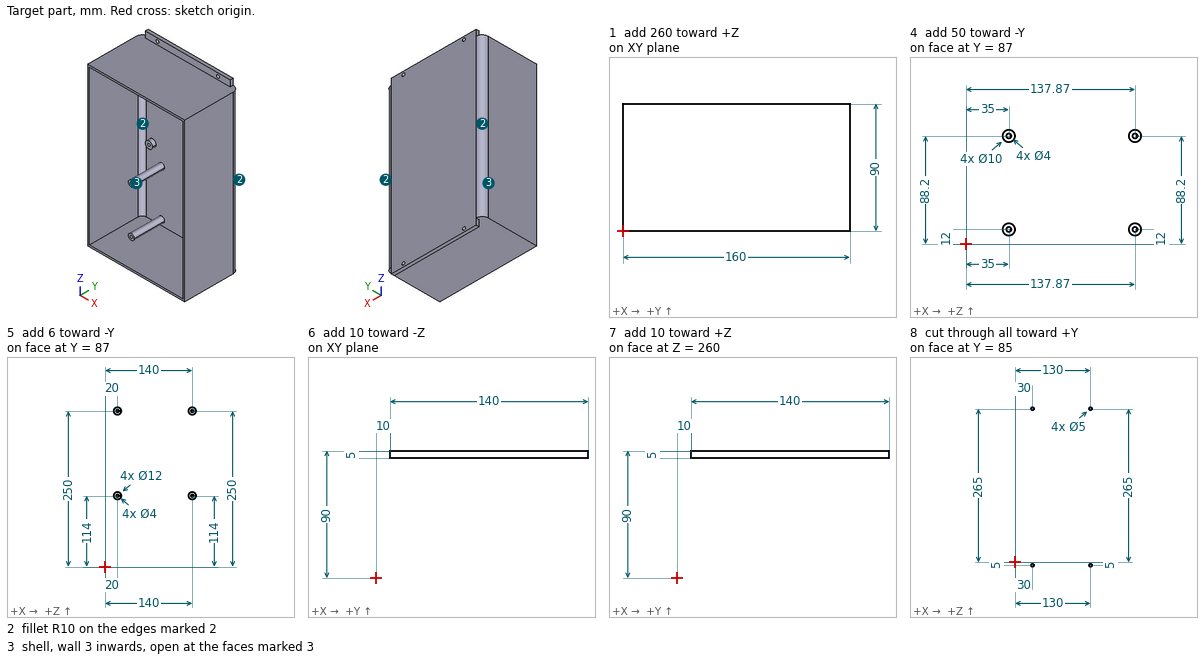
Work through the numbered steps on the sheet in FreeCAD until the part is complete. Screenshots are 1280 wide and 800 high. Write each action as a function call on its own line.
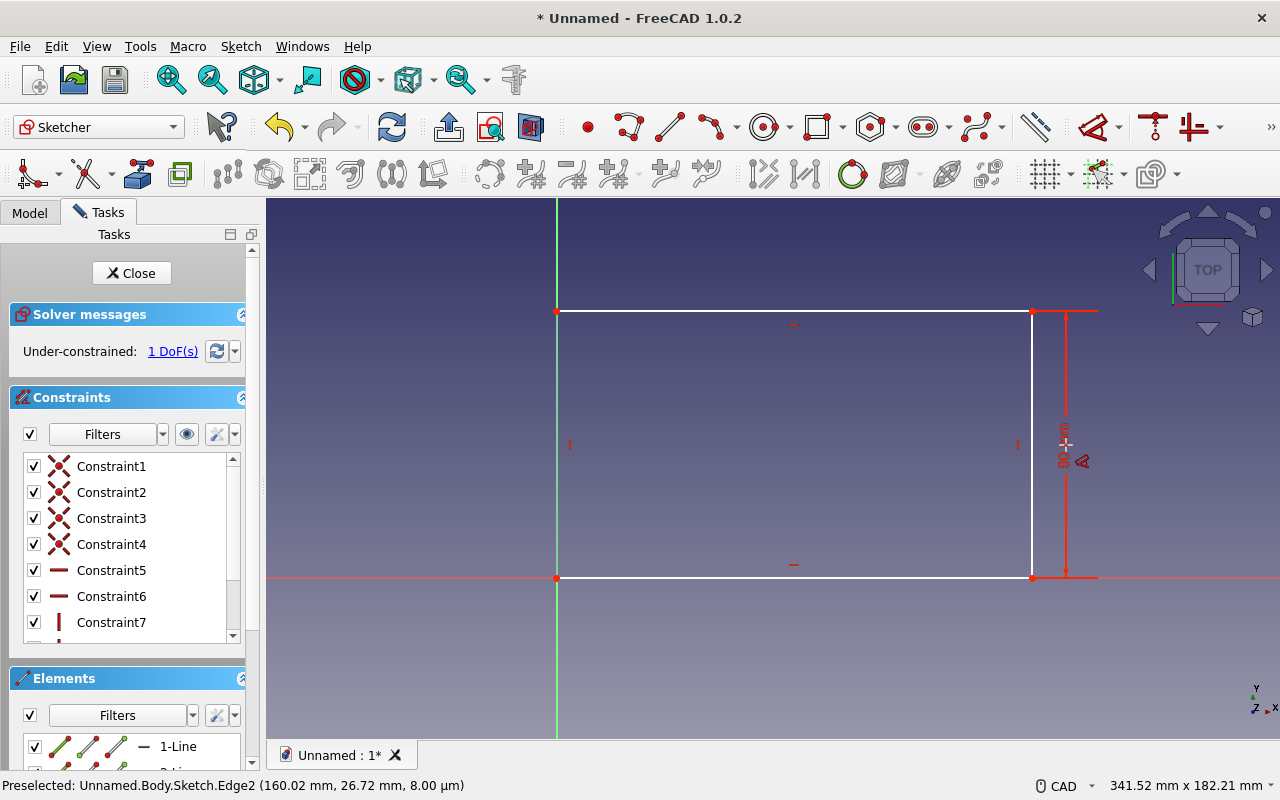
click(699, 578)
click(794, 612)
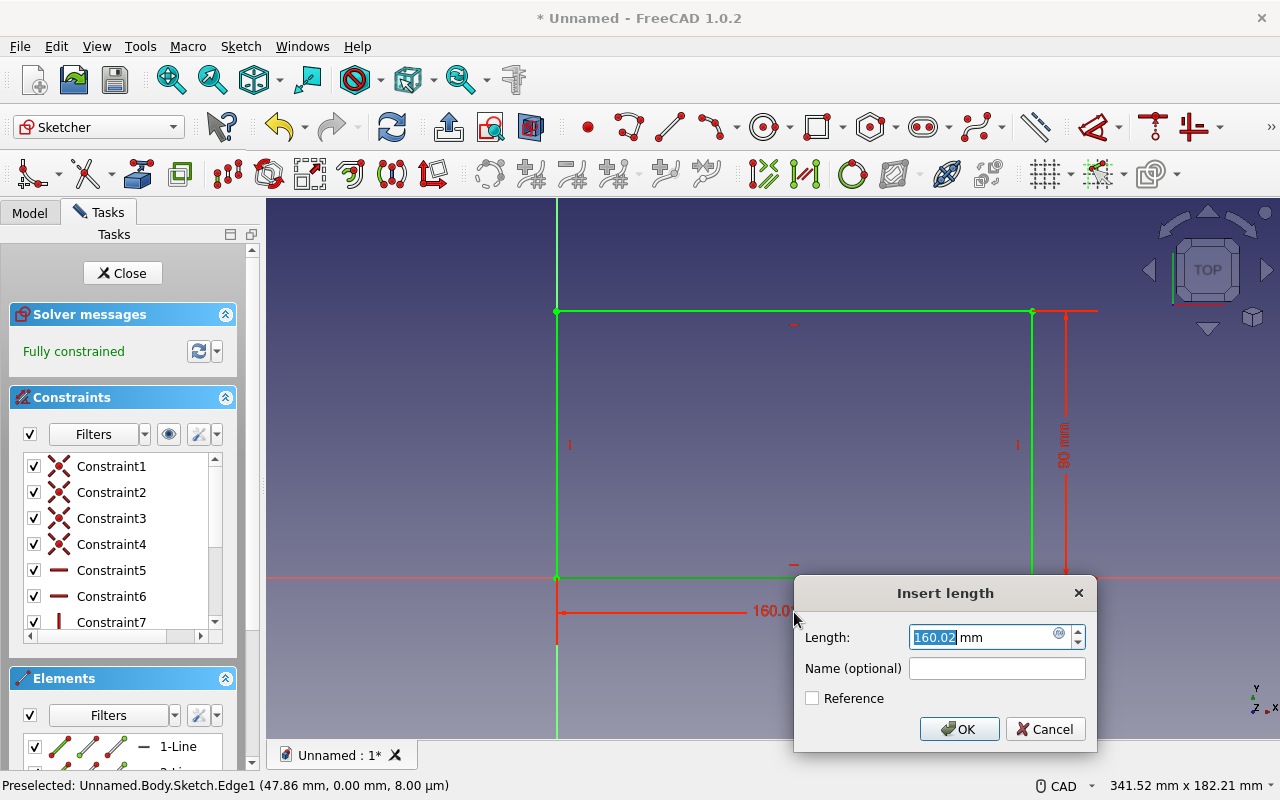
text(160)
key(Return)
key(Escape)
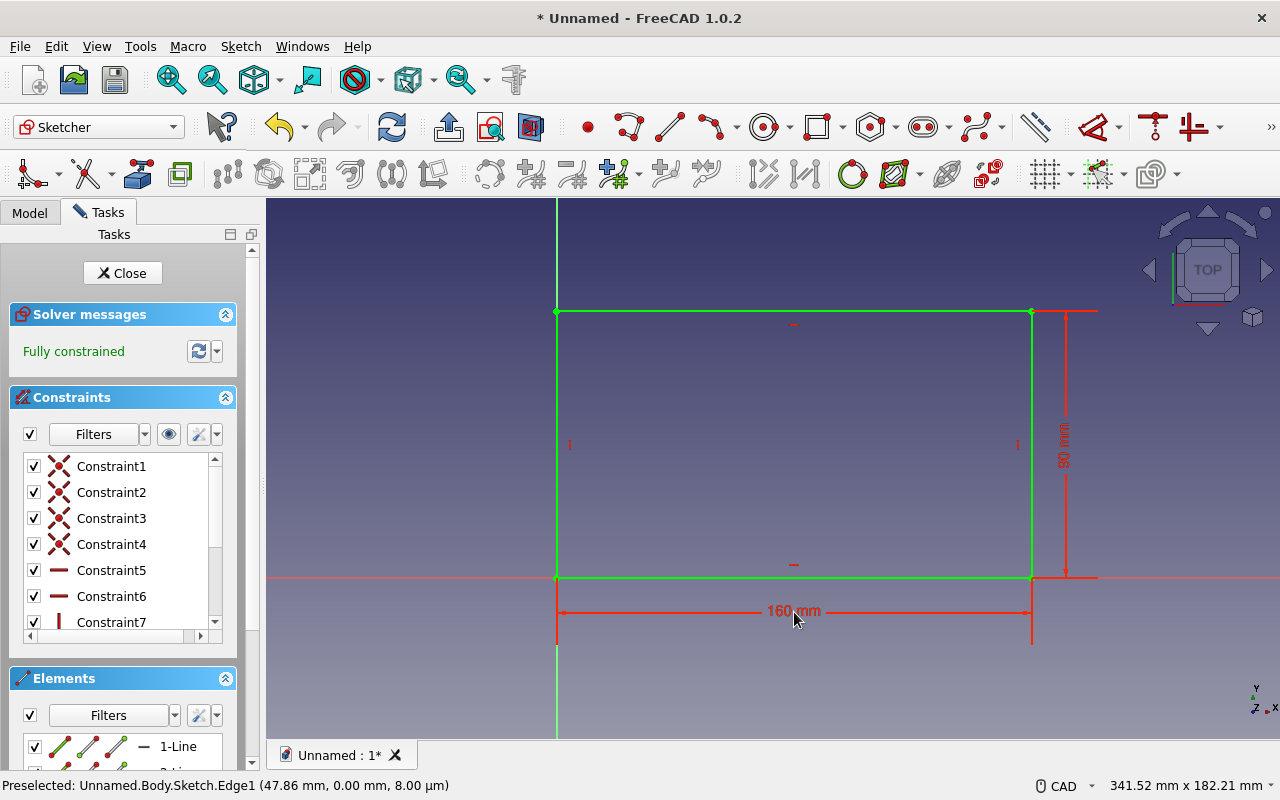
click(123, 273)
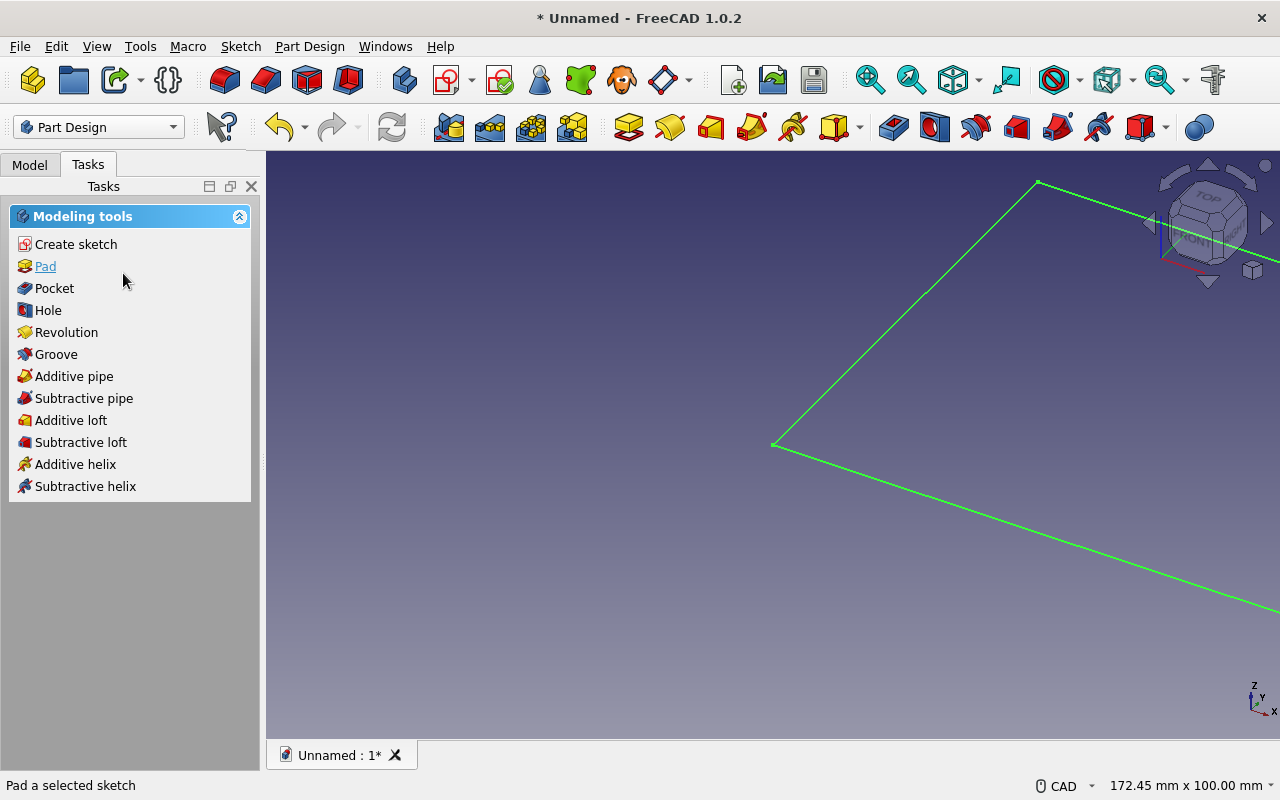
click(629, 128)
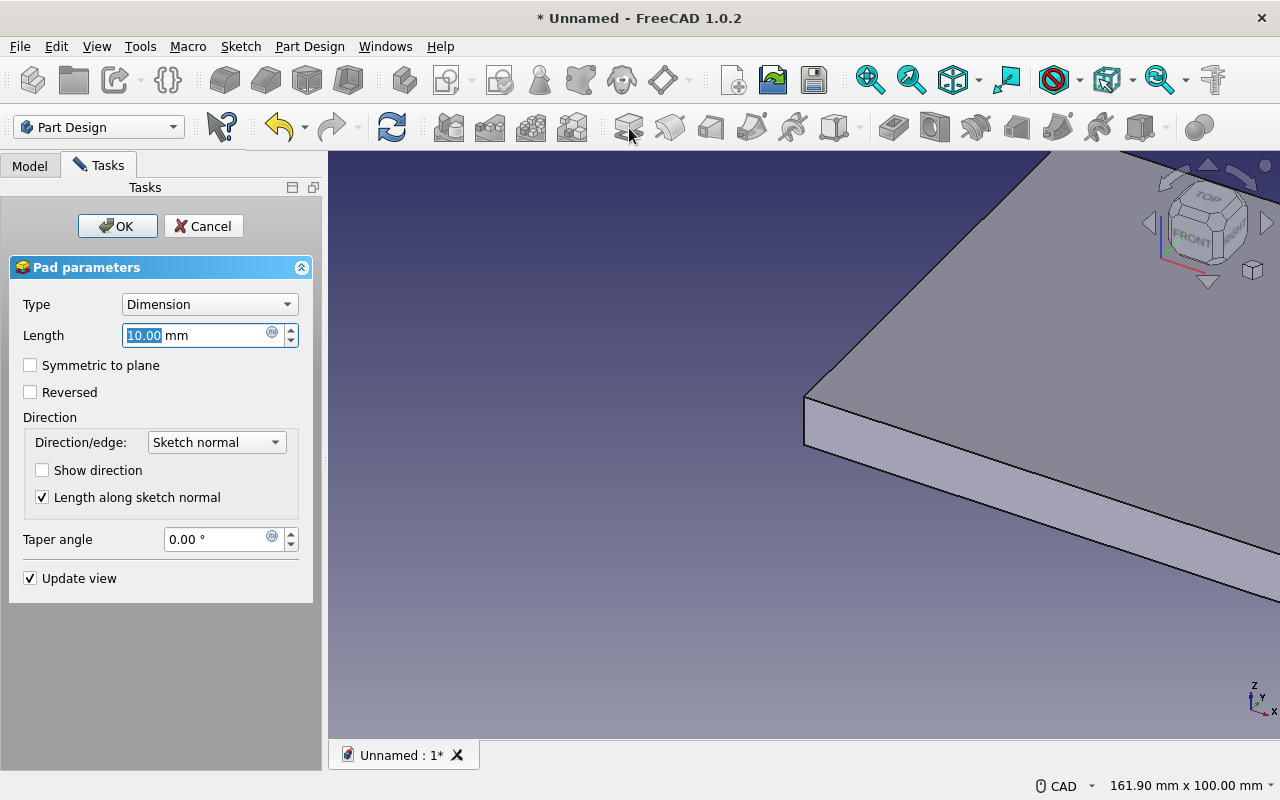
text(260)
key(Tab)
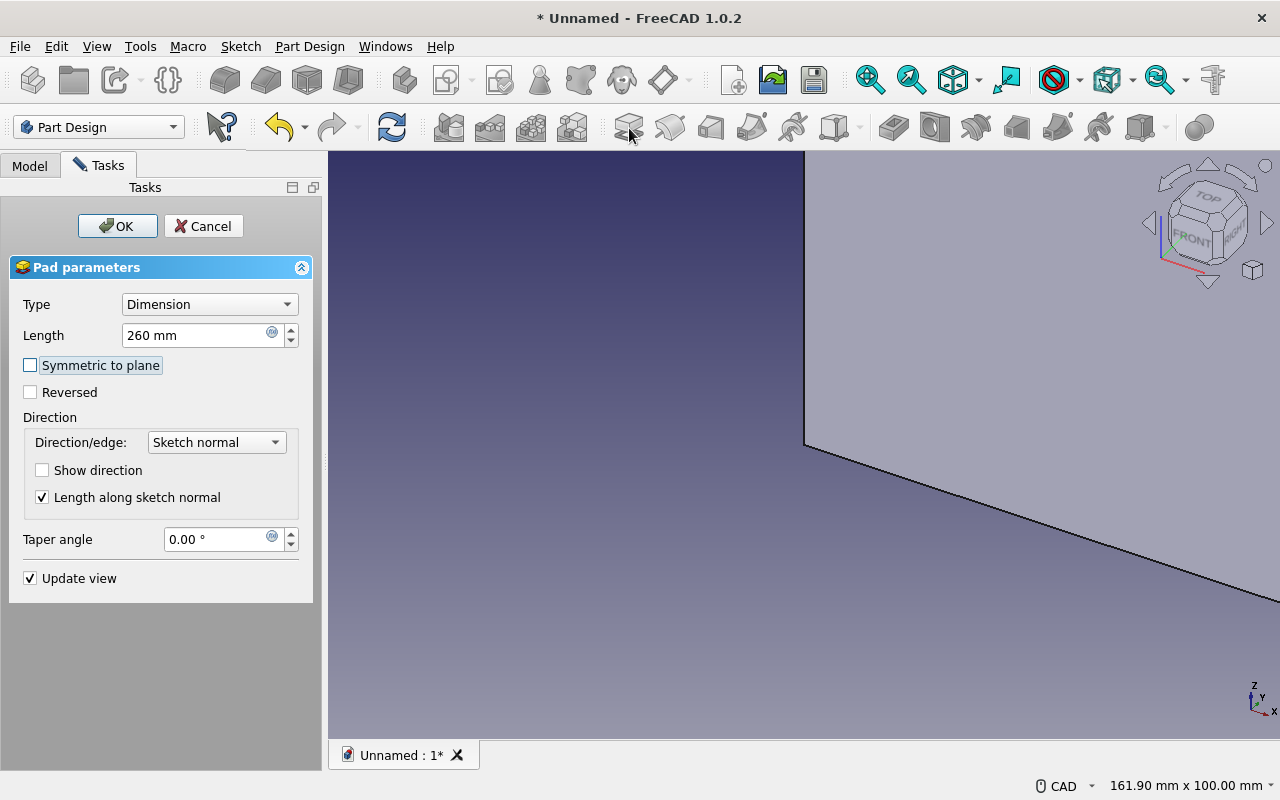
click(118, 226)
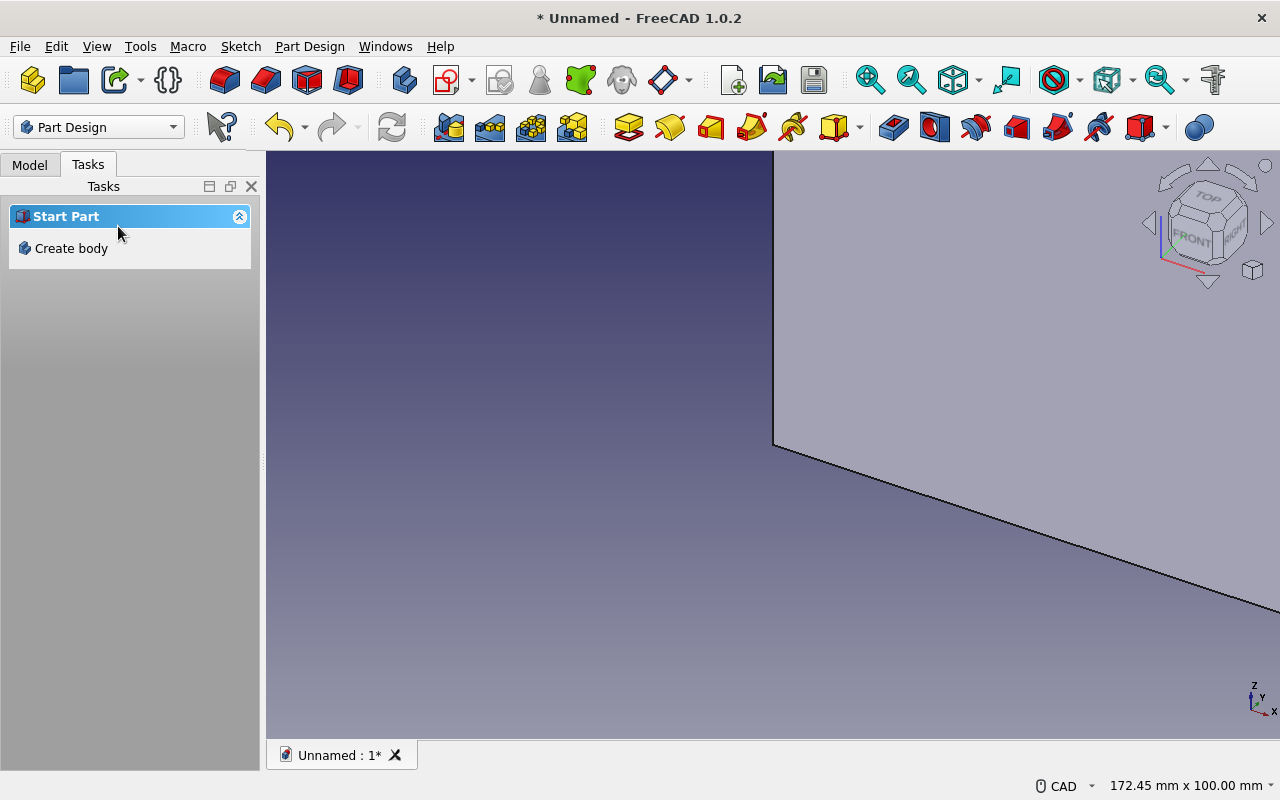
key(v)
key(f)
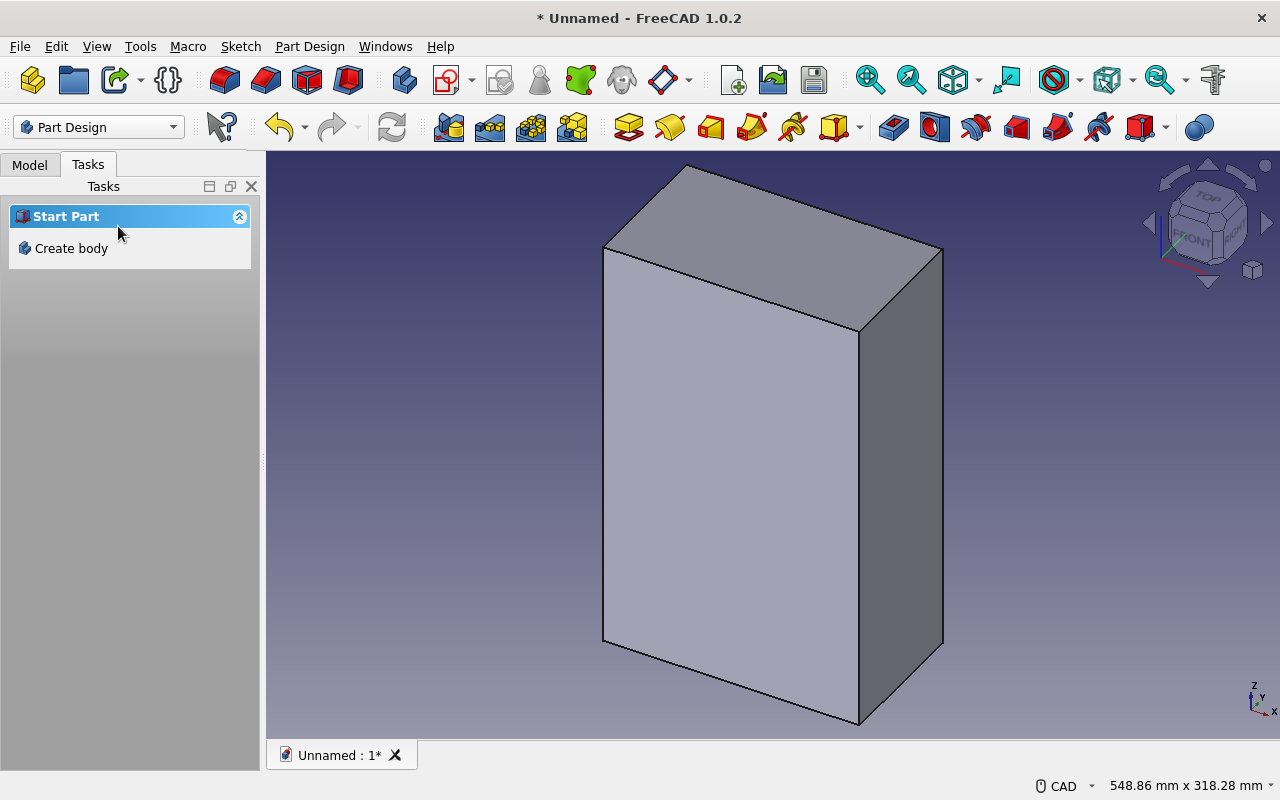
key(0)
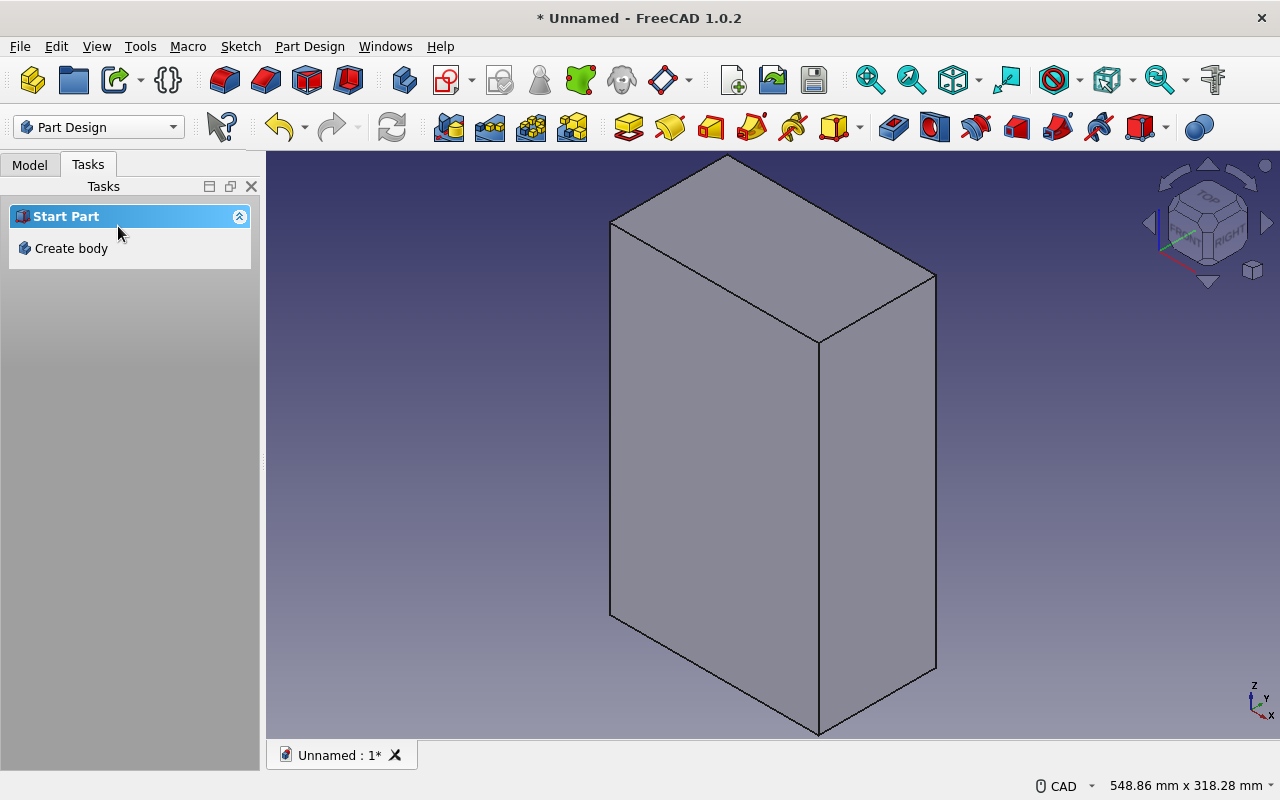
key(2)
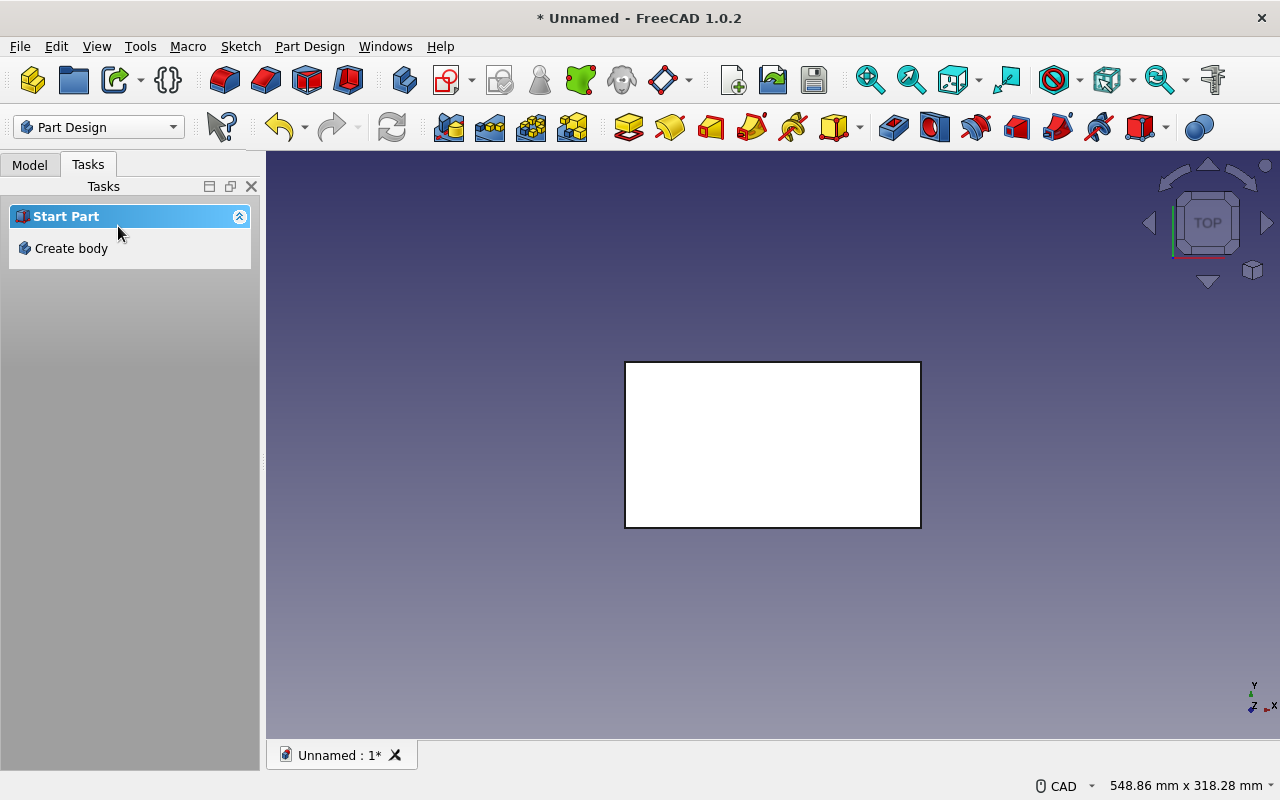
key(v)
key(f)